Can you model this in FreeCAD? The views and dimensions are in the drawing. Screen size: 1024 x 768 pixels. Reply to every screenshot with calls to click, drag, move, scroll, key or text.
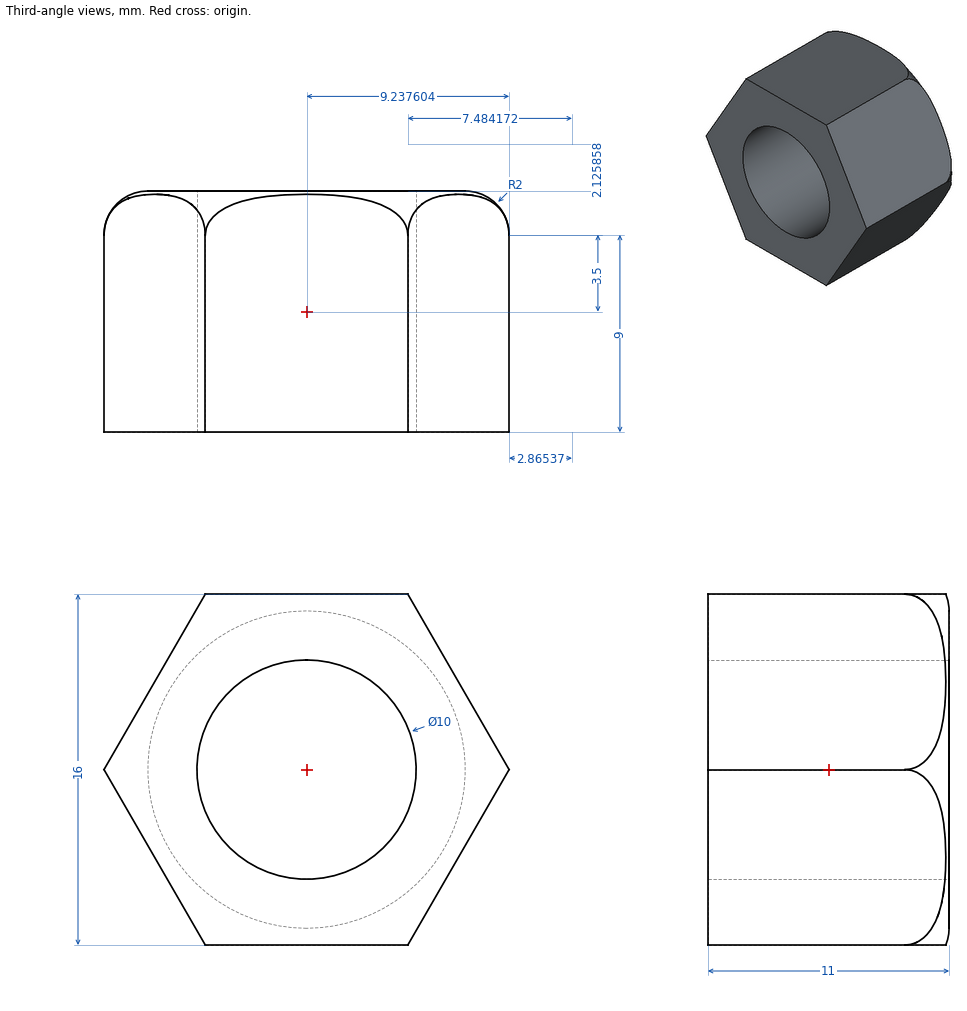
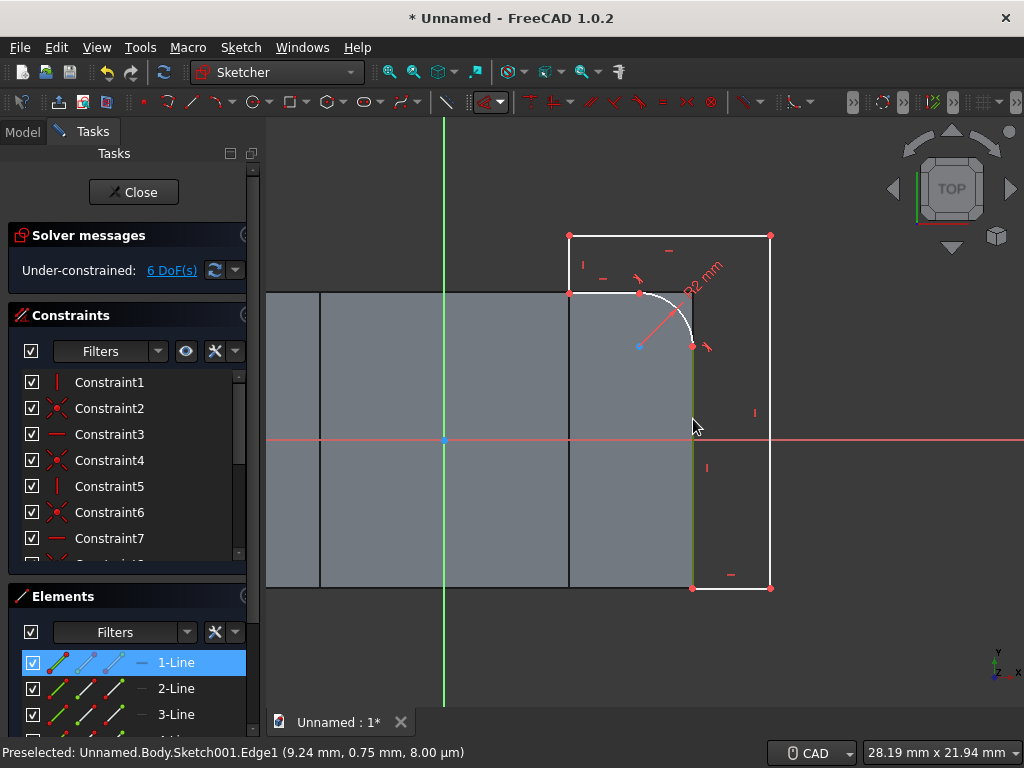
click(502, 102)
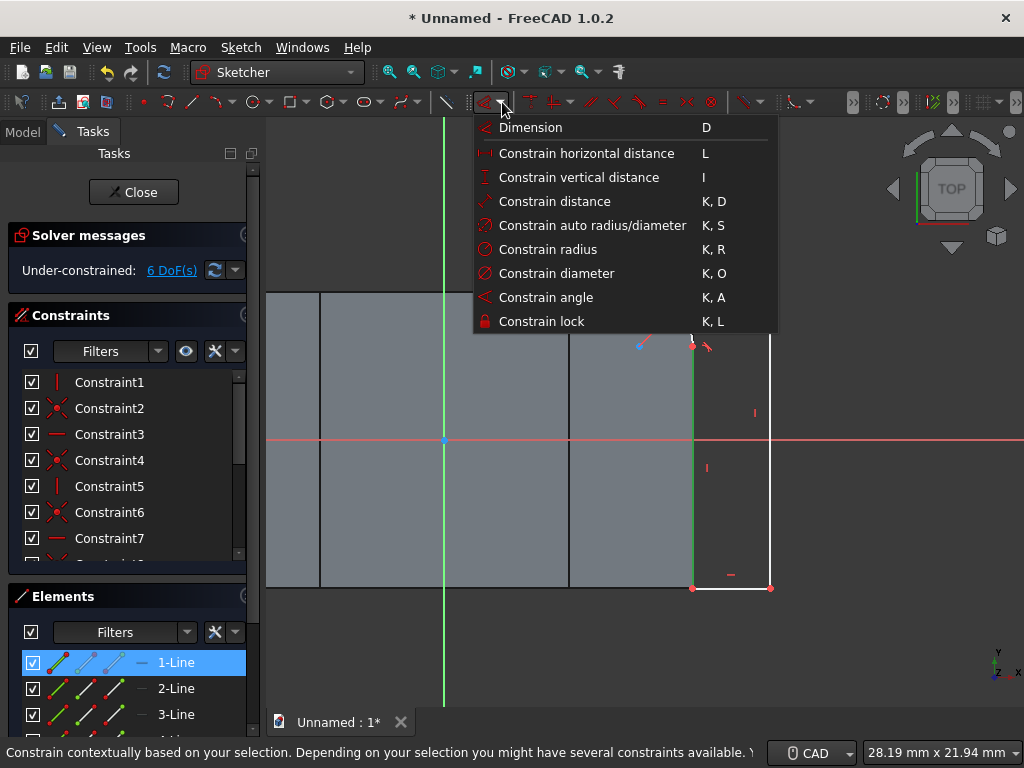
click(626, 177)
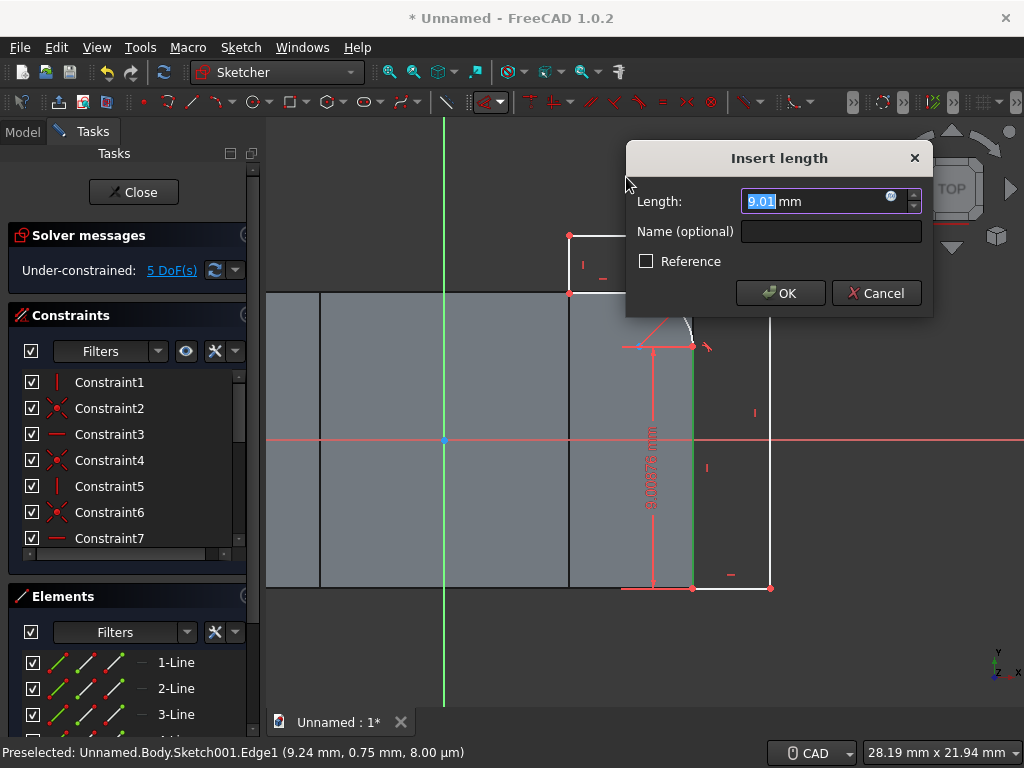
text(9)
key(Return)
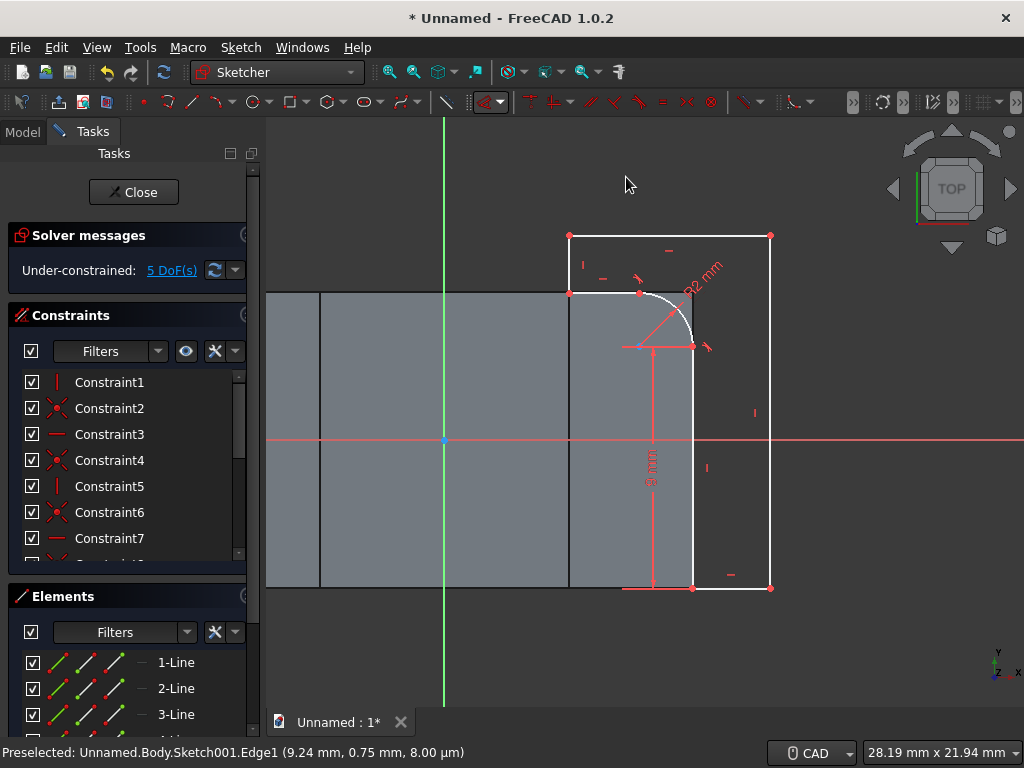
click(693, 347)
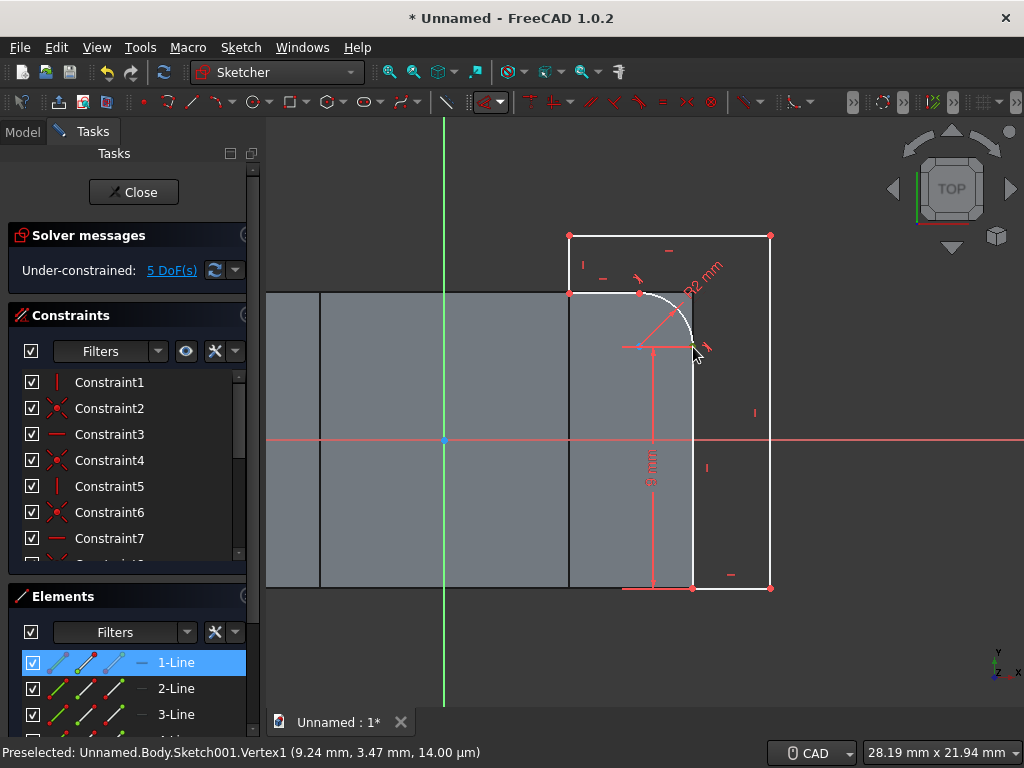
click(502, 102)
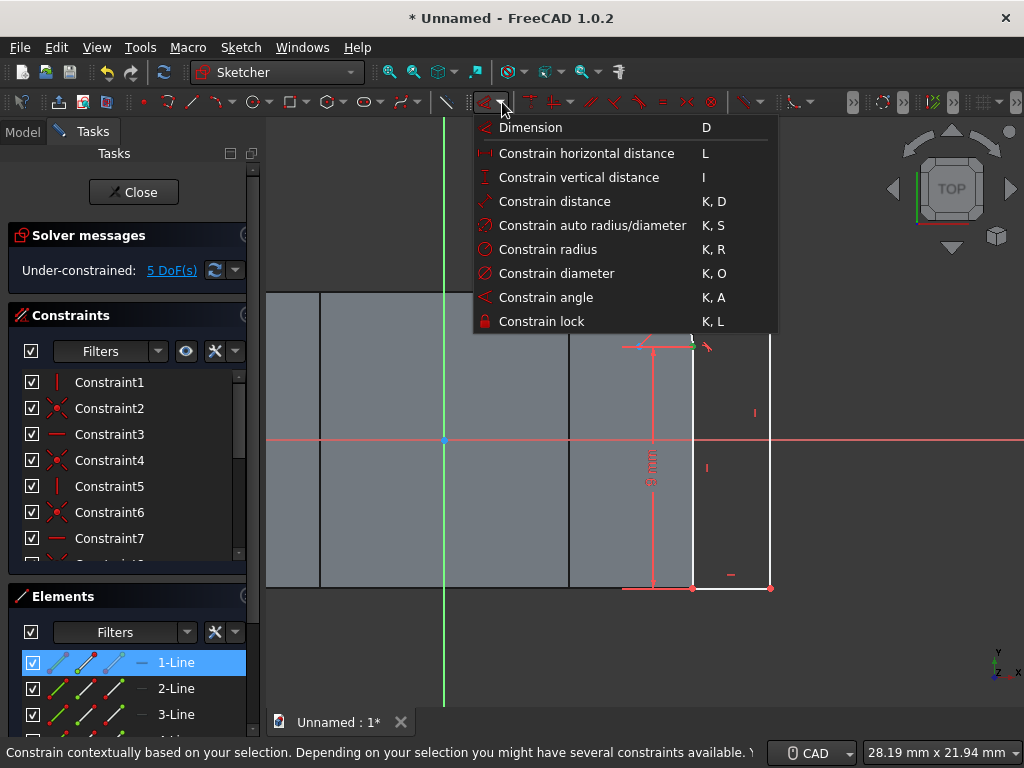
click(626, 177)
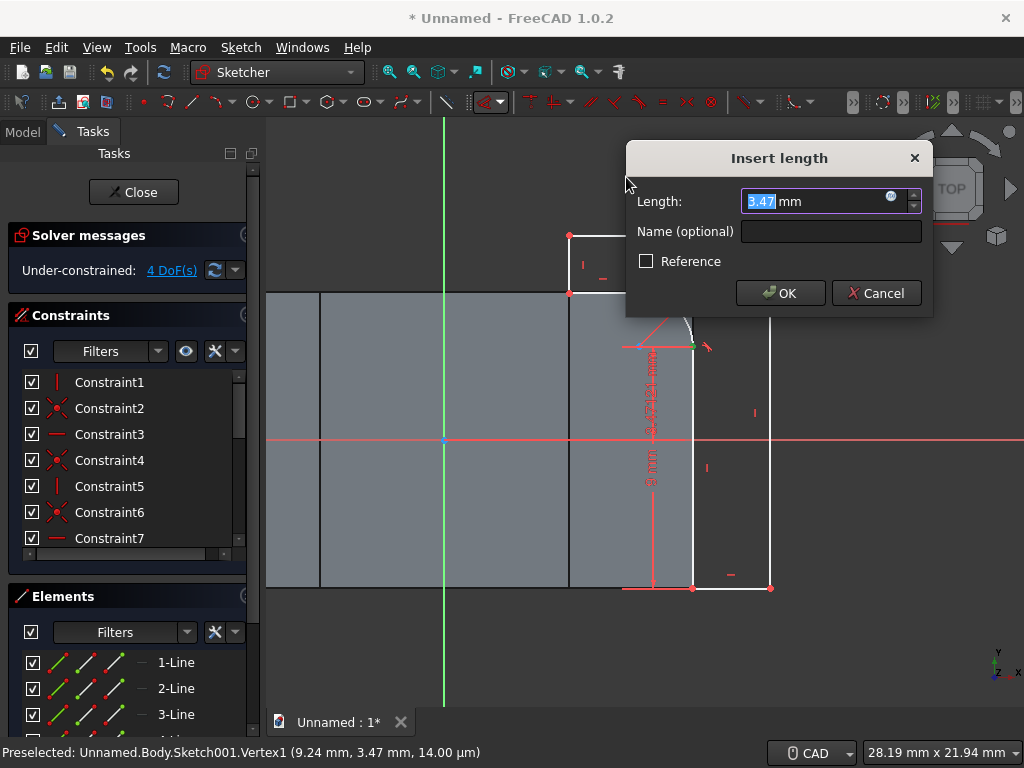
text(3.5)
key(Return)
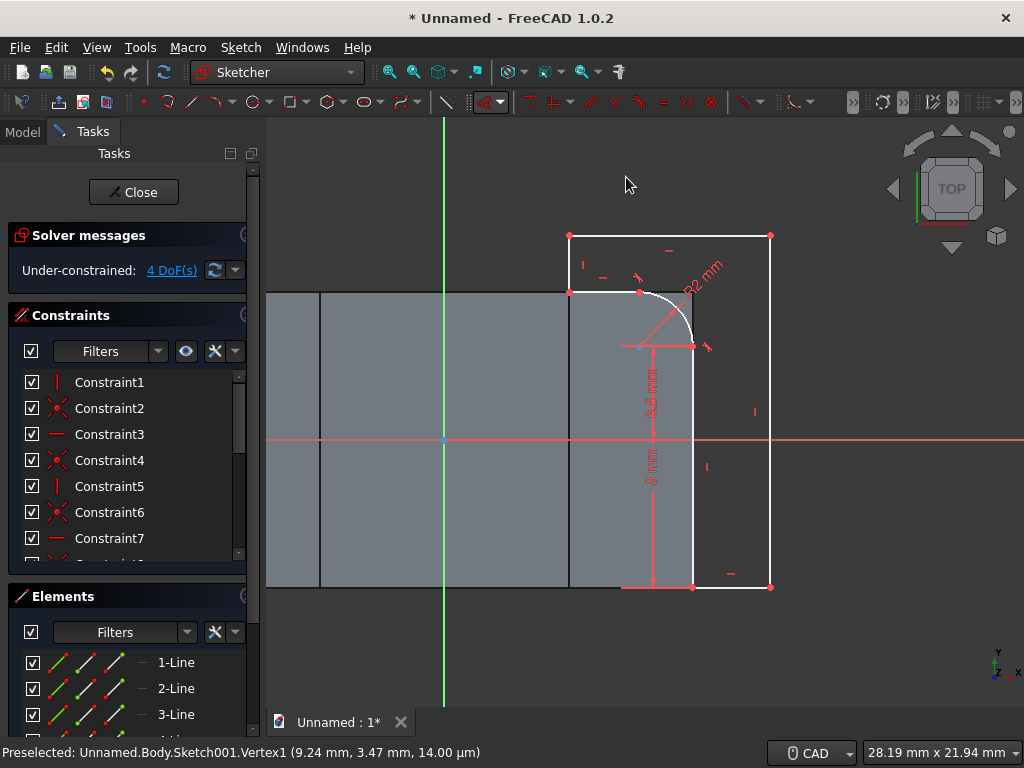
click(716, 588)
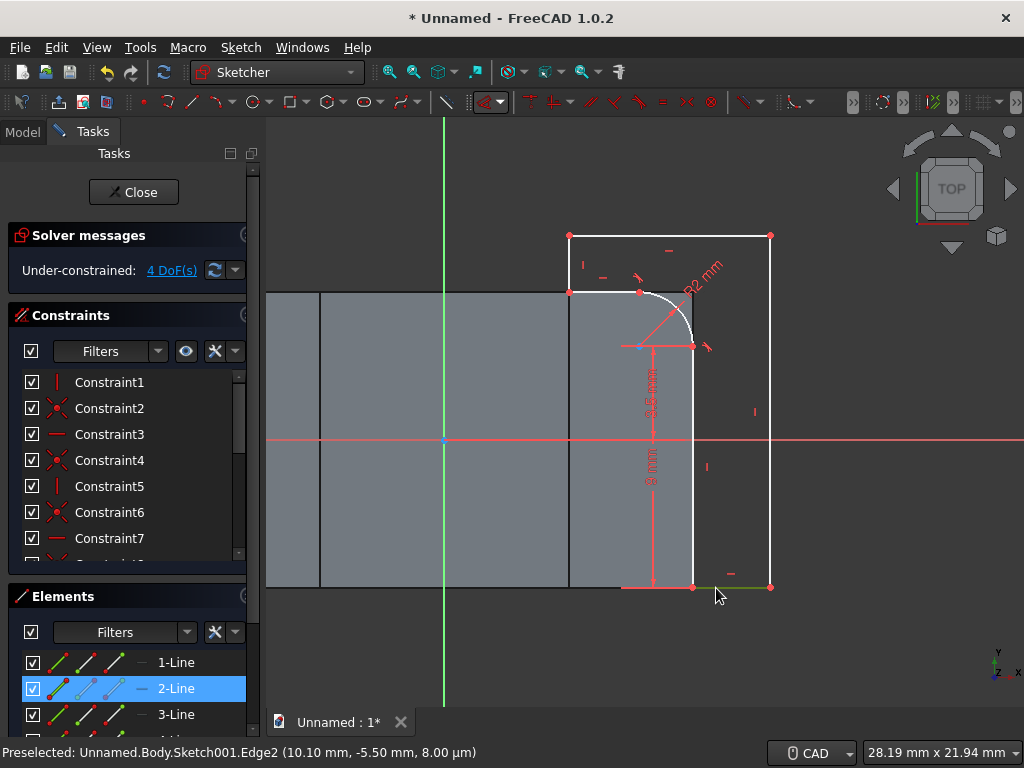
key(l)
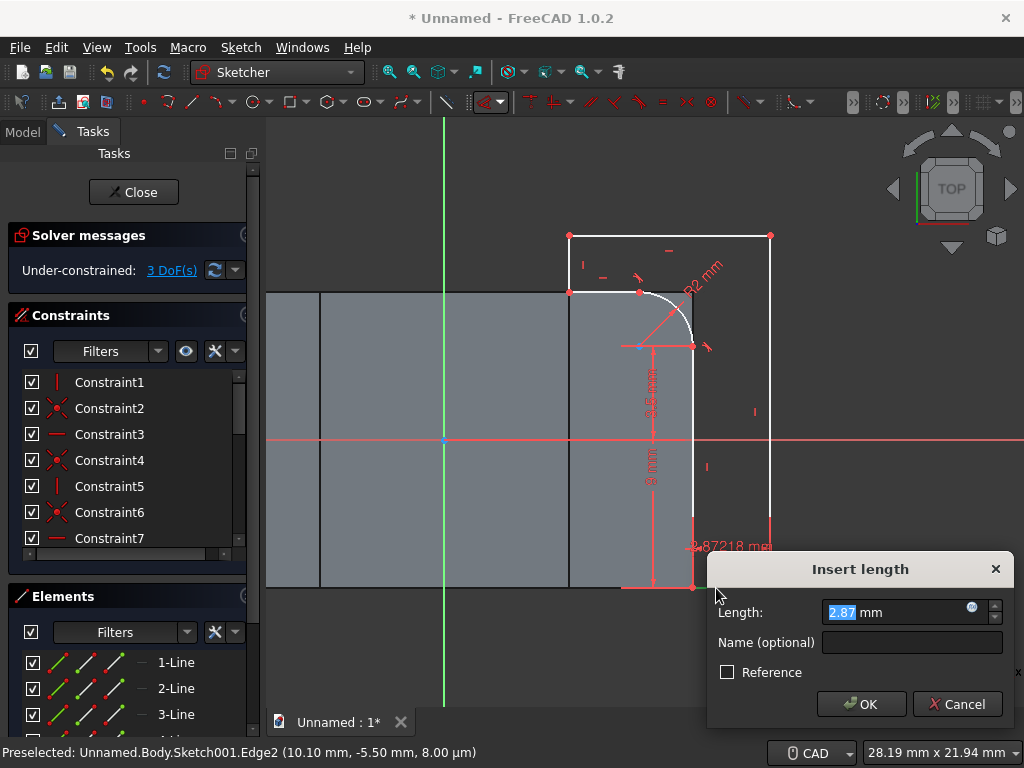
text(2.86537)
key(Return)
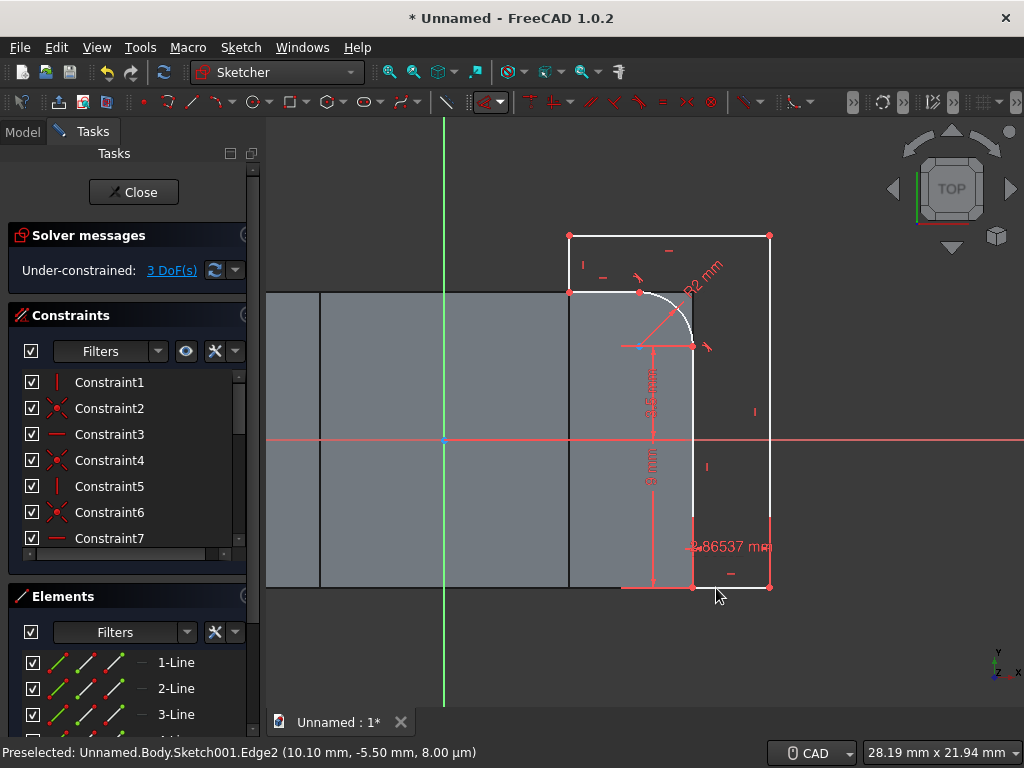
click(710, 236)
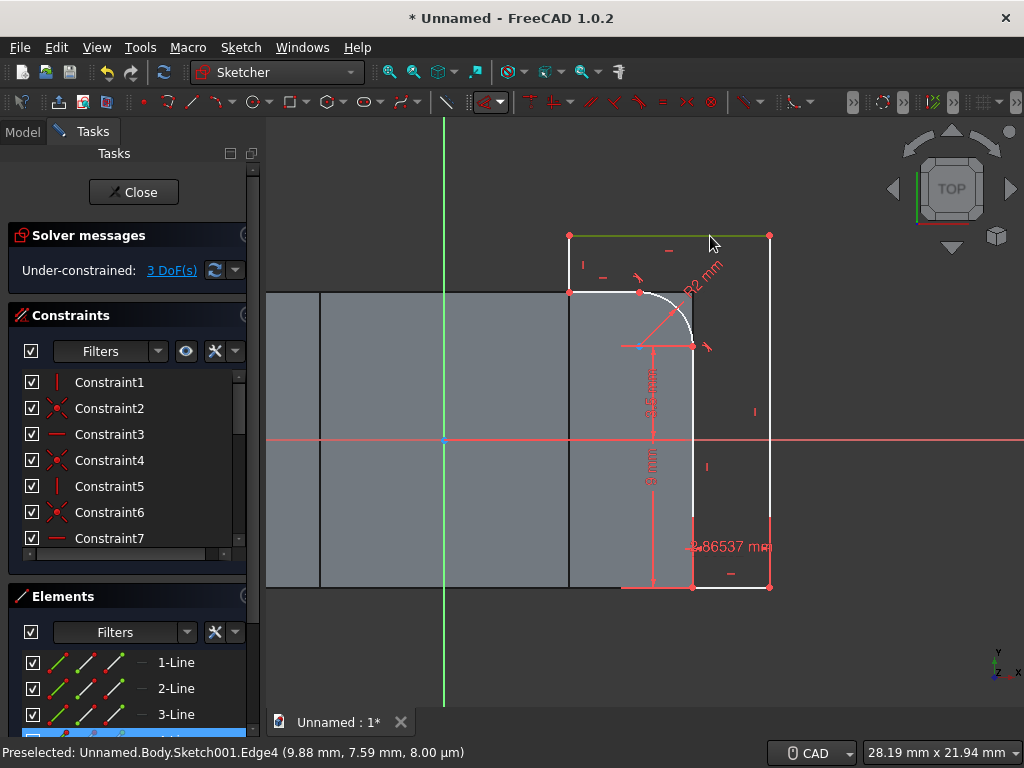
key(l)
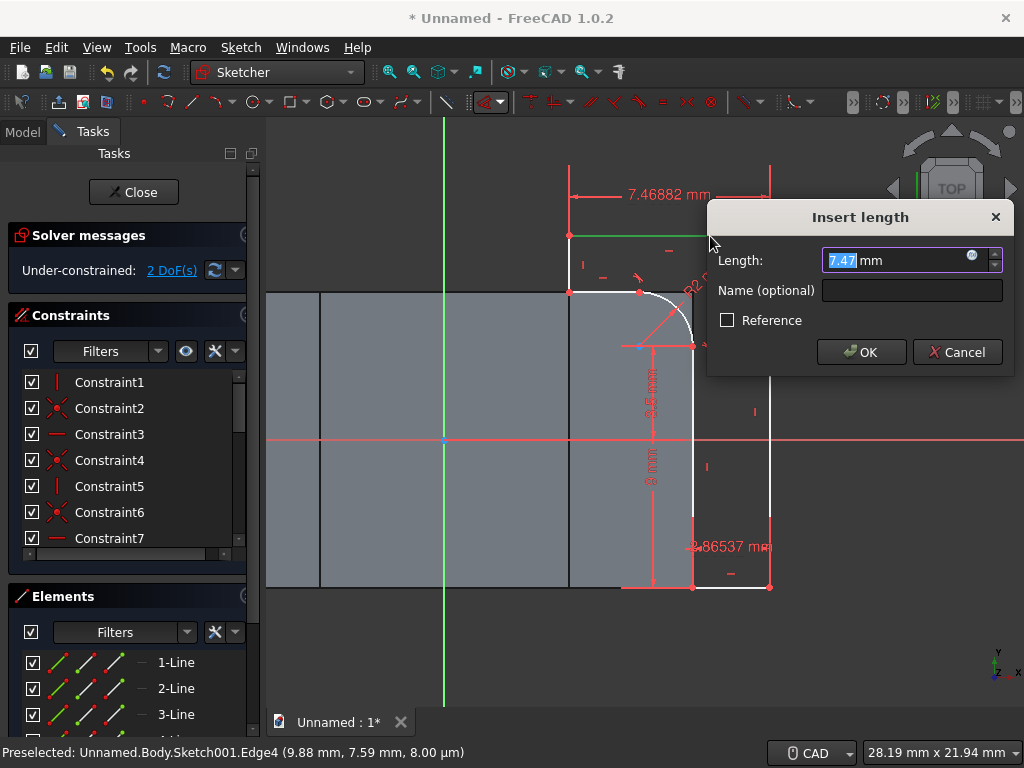
text(7.484172)
key(Return)